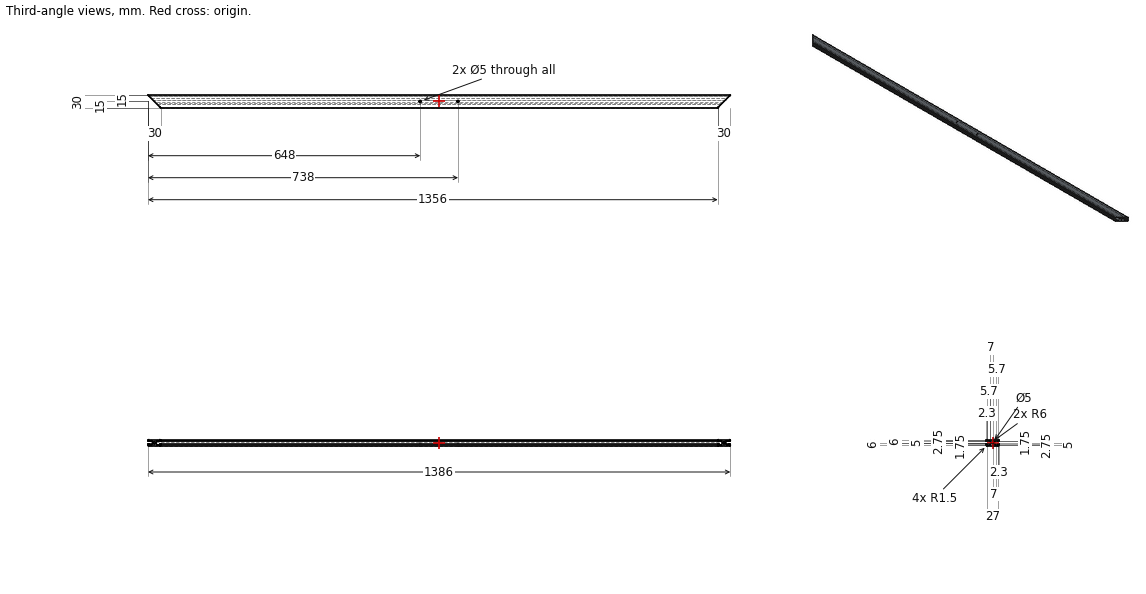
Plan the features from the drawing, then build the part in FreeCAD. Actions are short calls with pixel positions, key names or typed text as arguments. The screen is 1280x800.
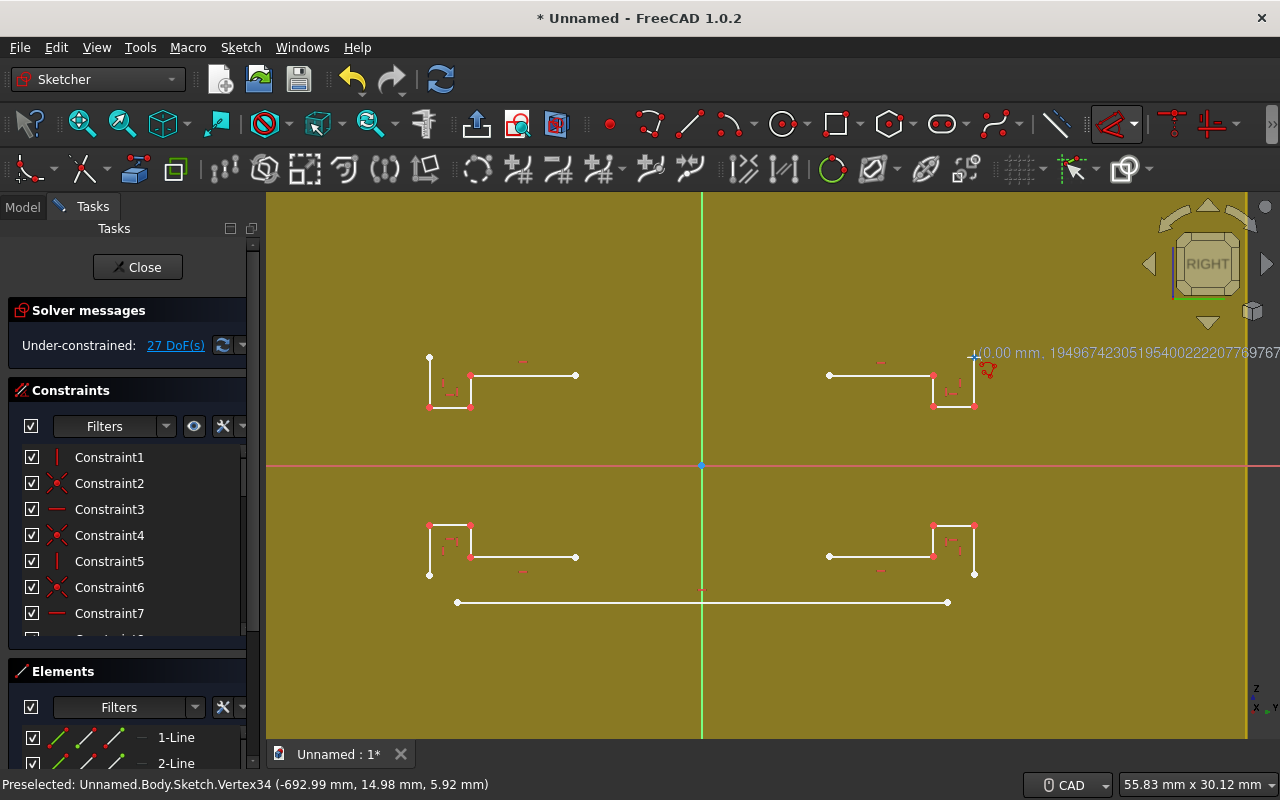
click(690, 124)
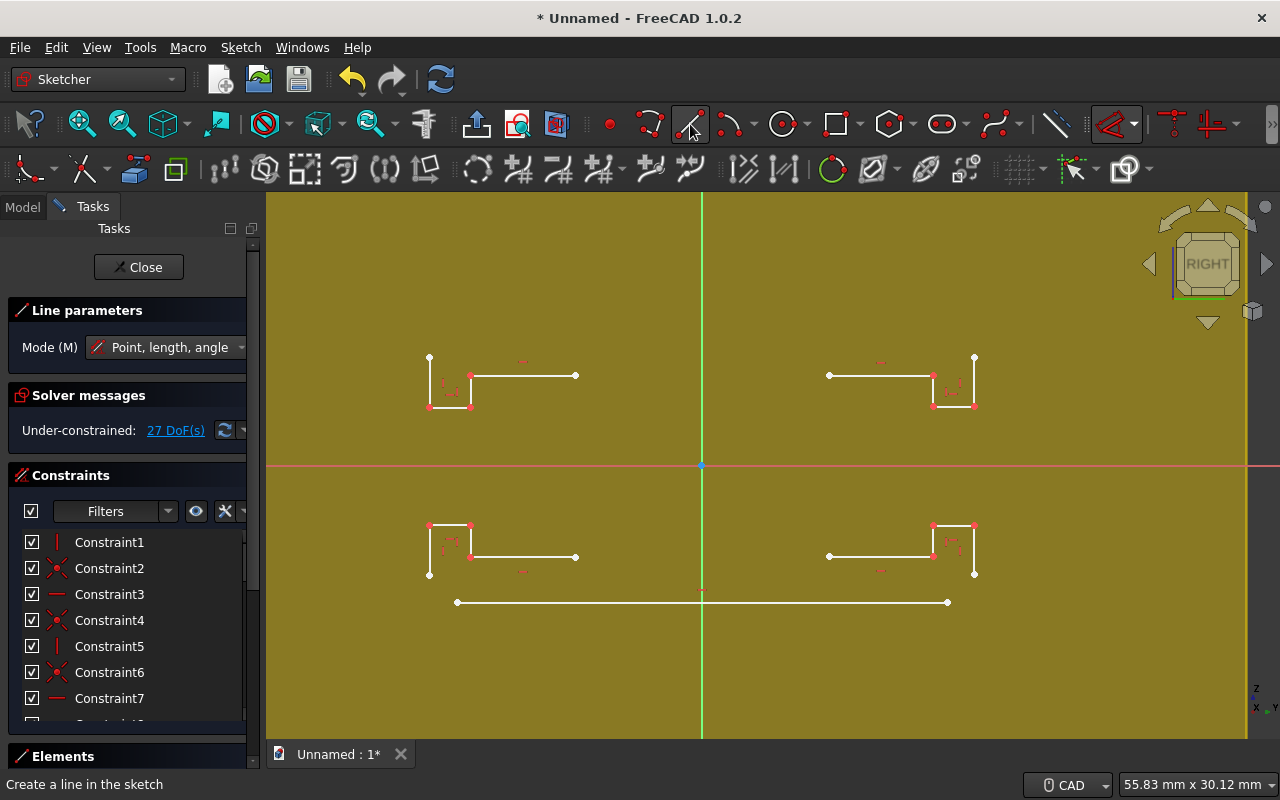
click(947, 329)
click(457, 329)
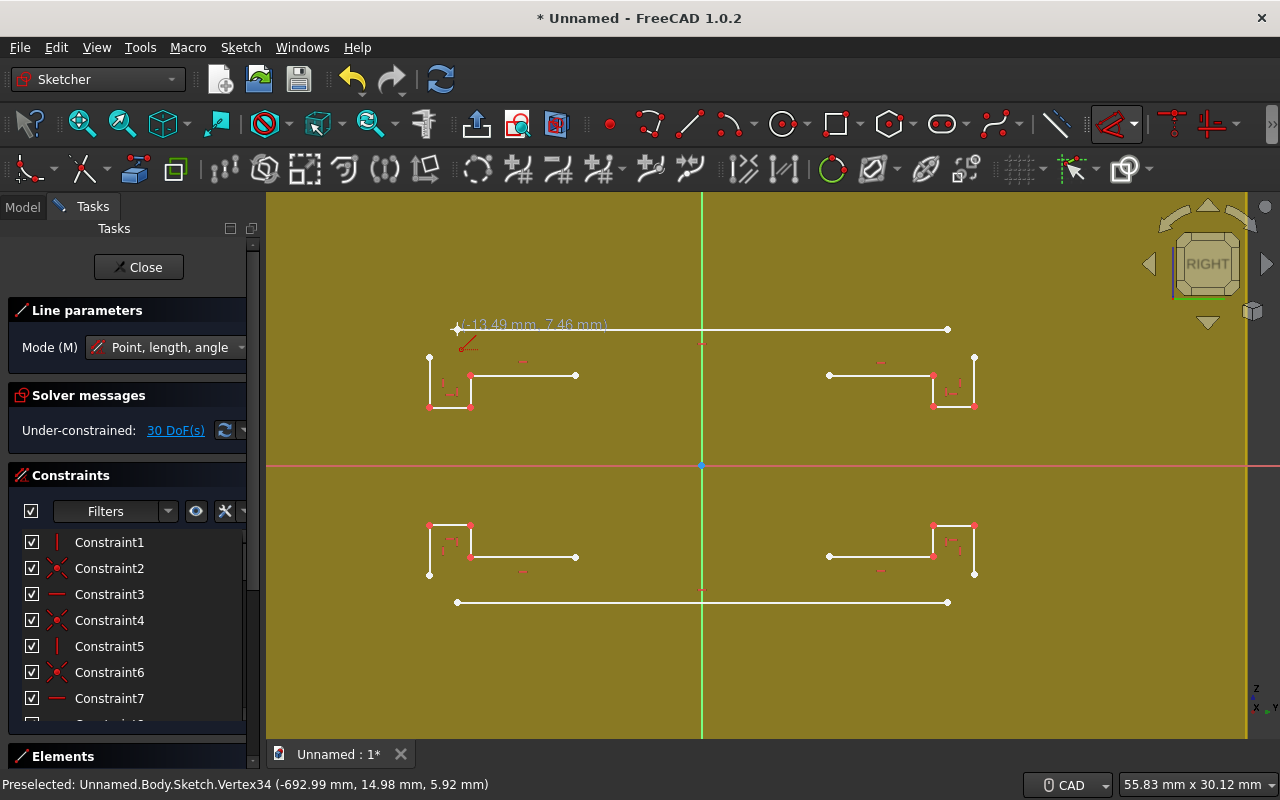
key(g)
key(3)
key(a)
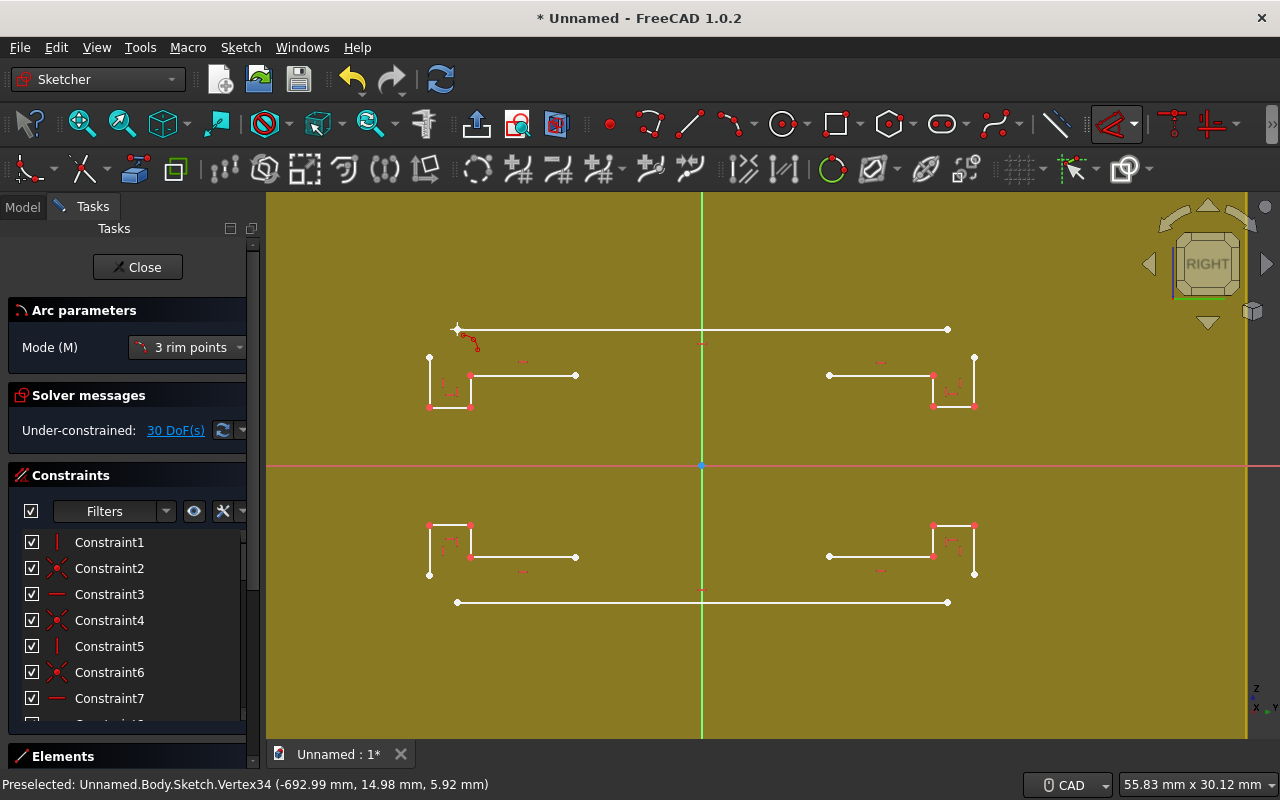
click(575, 376)
click(575, 557)
click(621, 487)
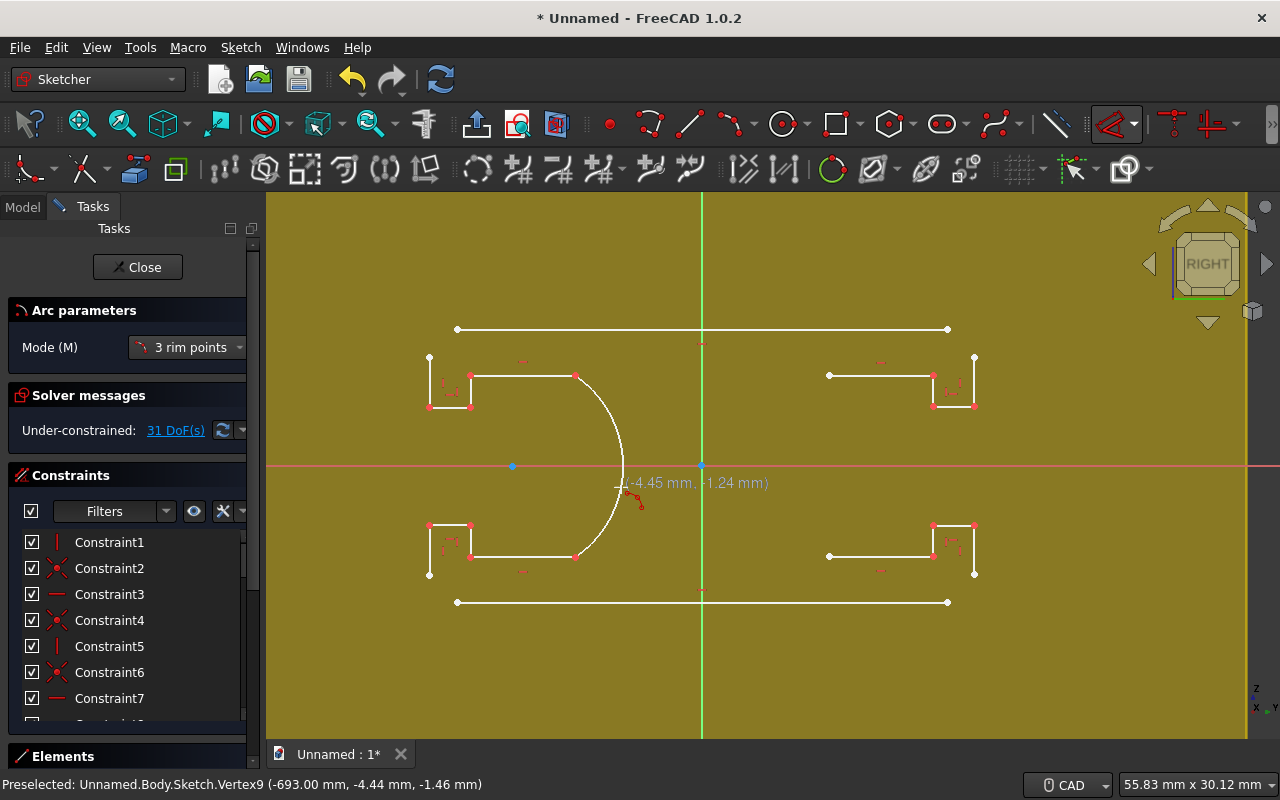
click(430, 575)
click(457, 603)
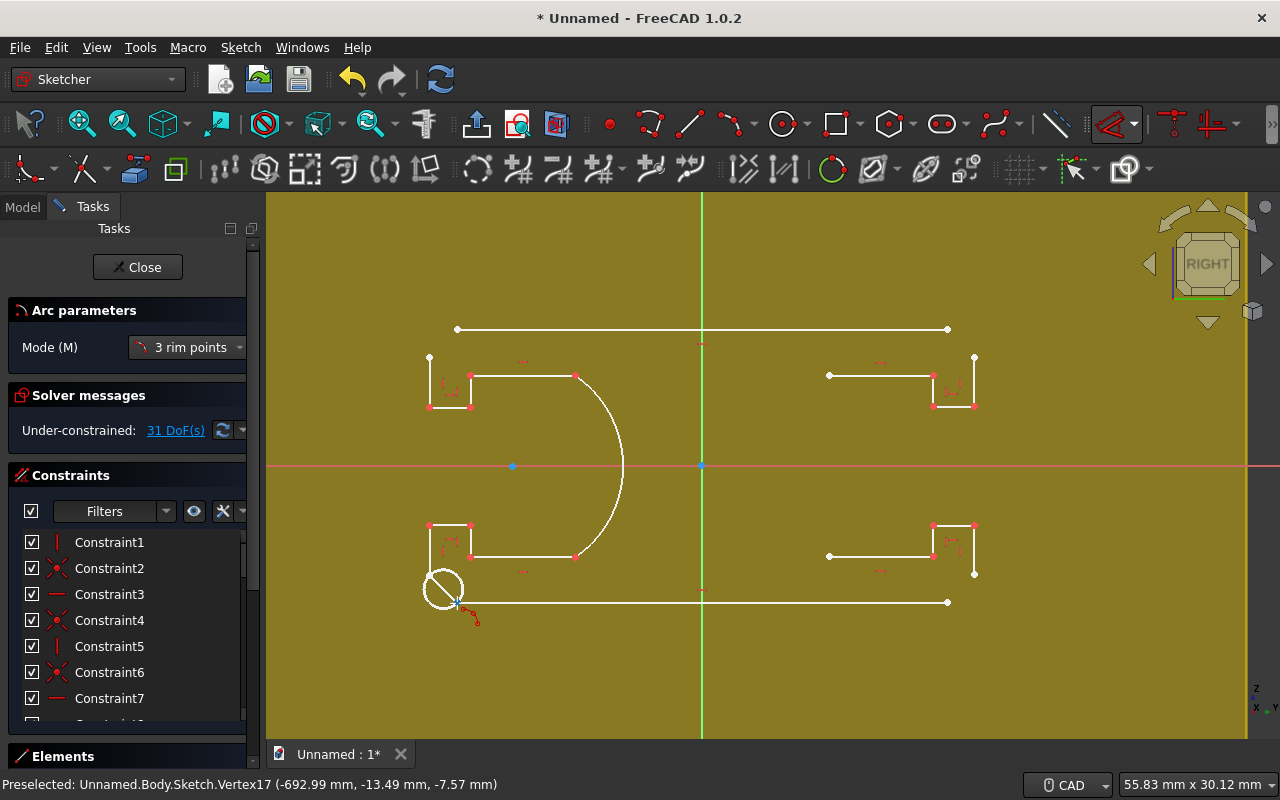
scroll(437, 594, up, 4)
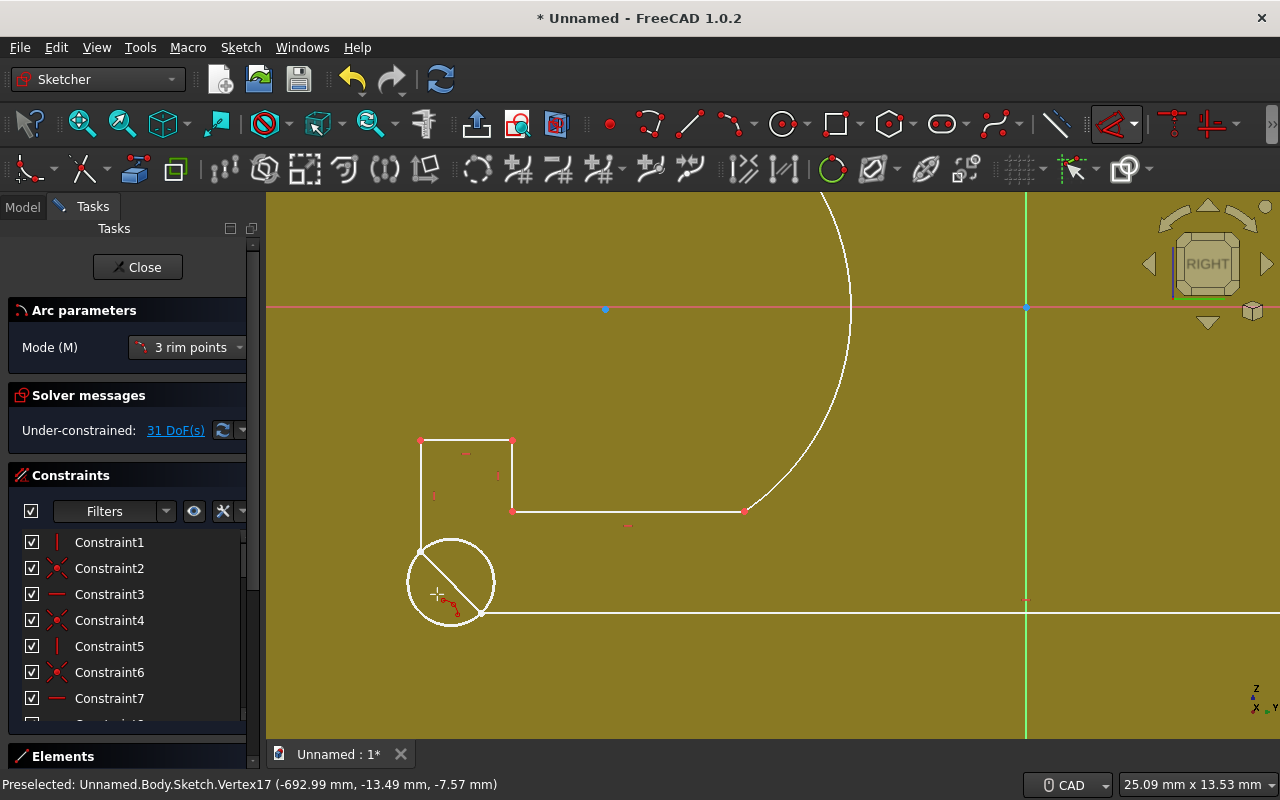
click(438, 592)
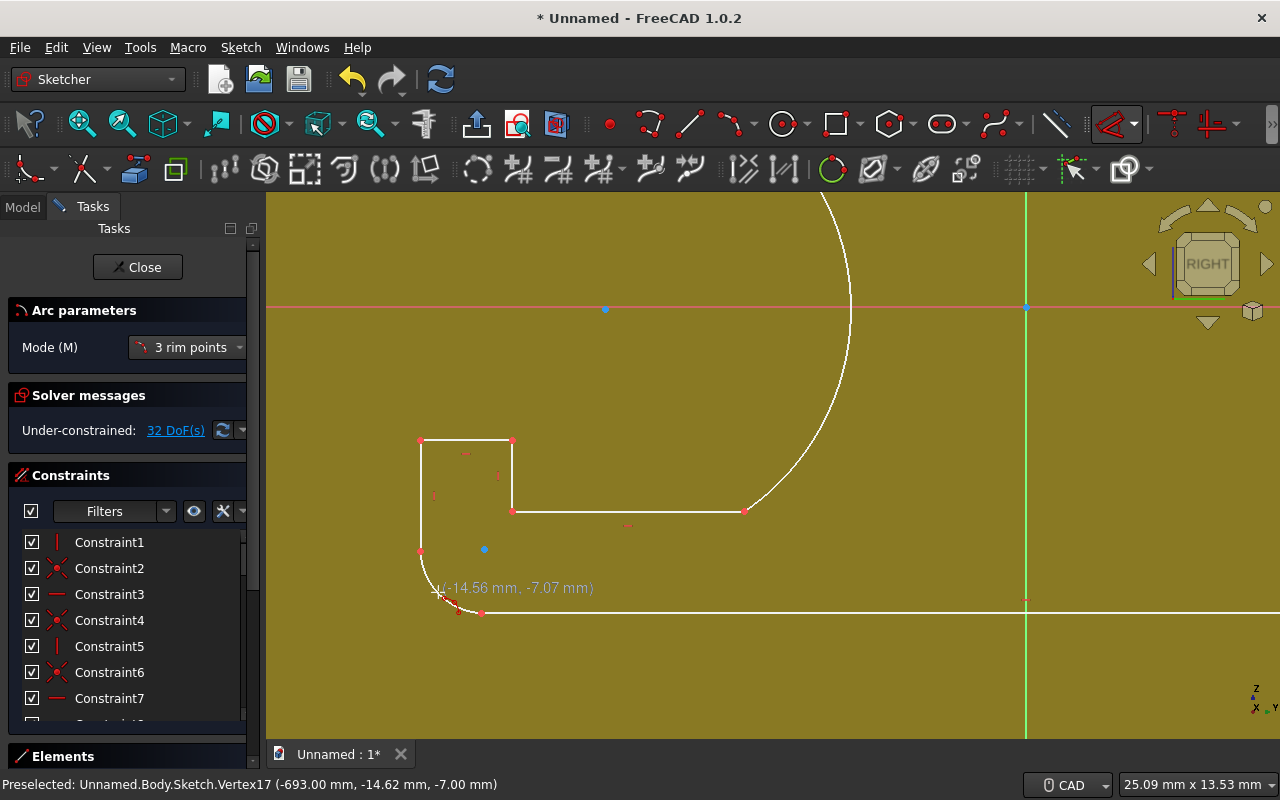
scroll(442, 595, down, 4)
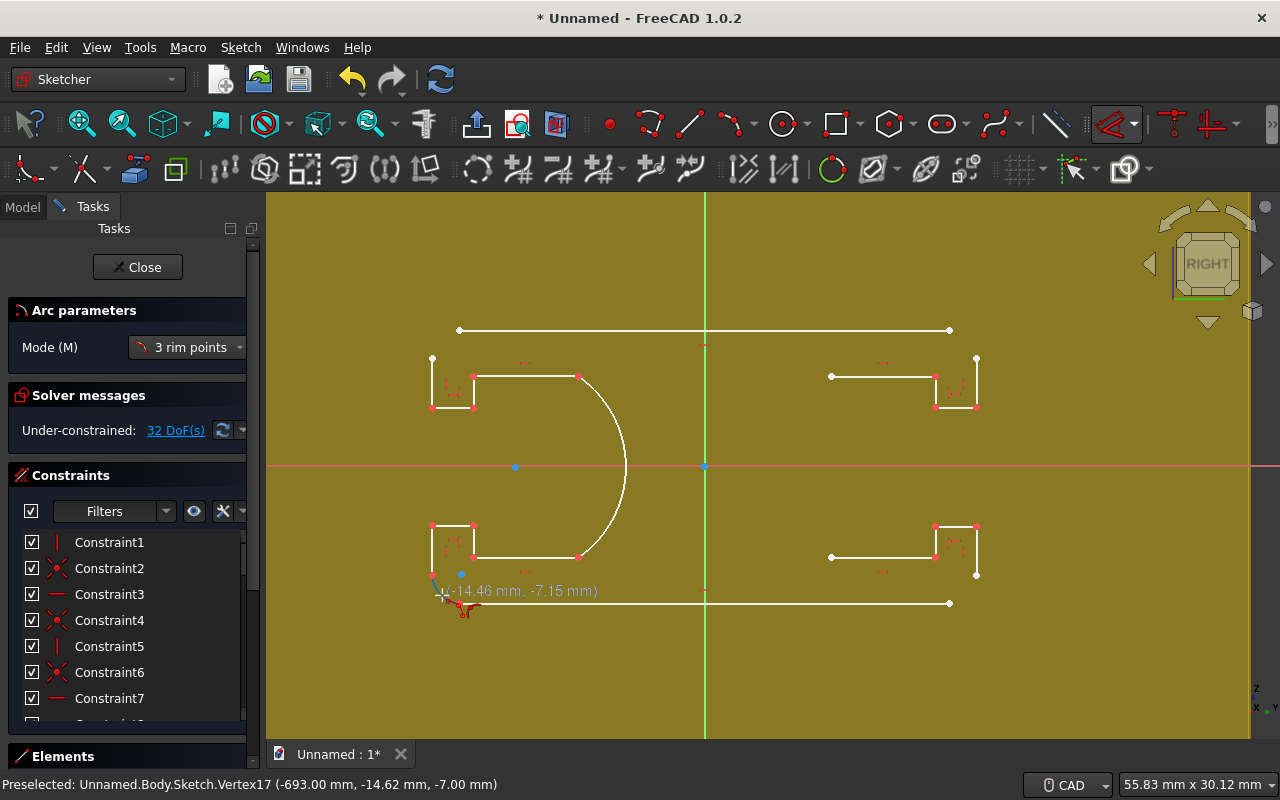
click(950, 604)
click(977, 576)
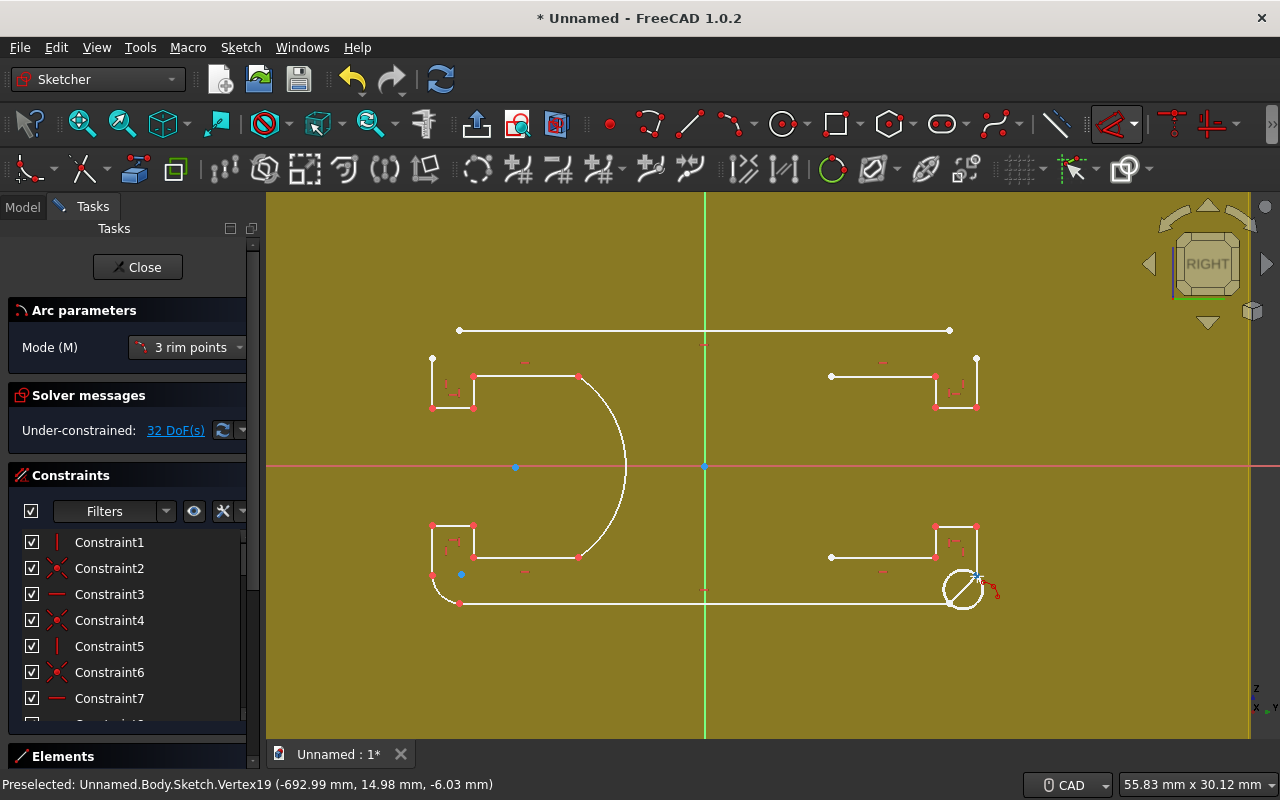
scroll(969, 594, up, 4)